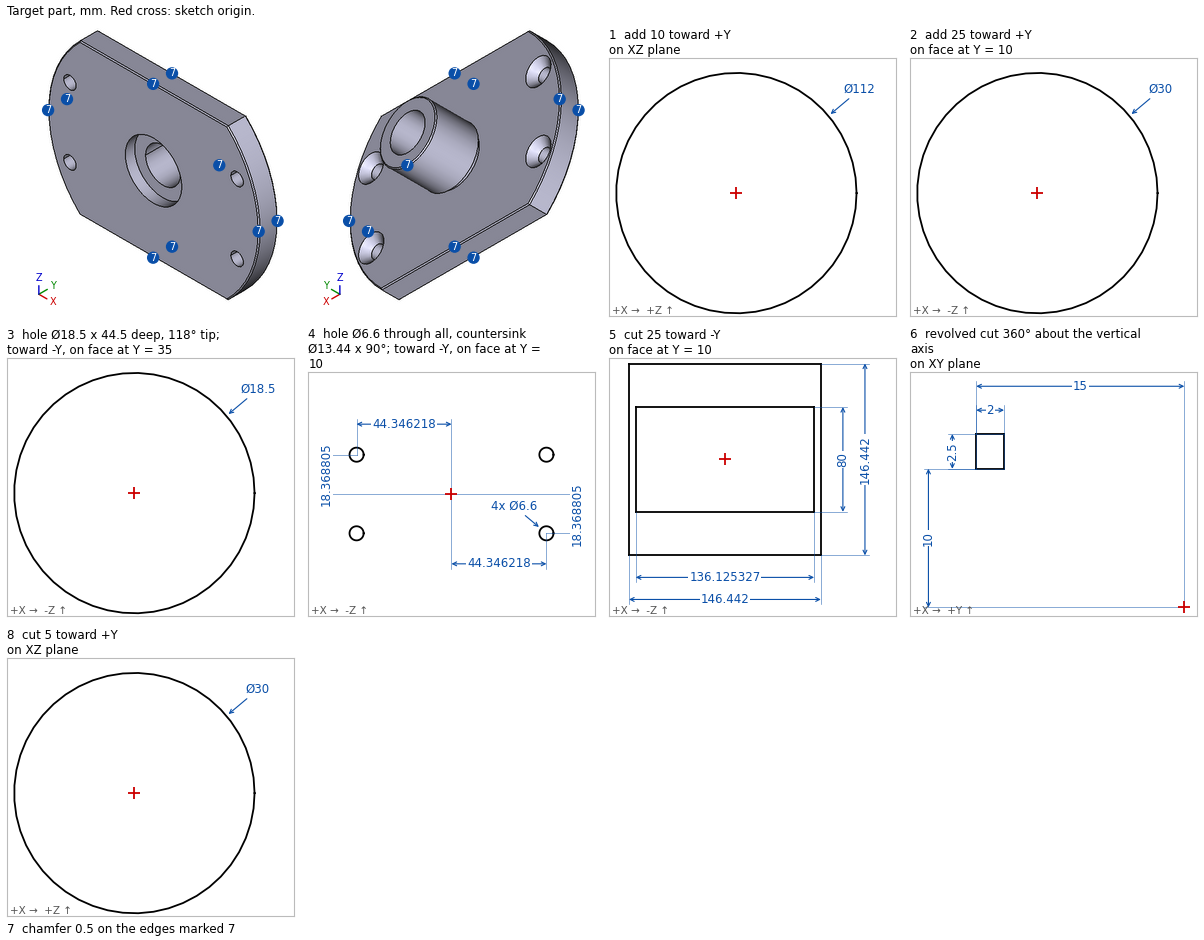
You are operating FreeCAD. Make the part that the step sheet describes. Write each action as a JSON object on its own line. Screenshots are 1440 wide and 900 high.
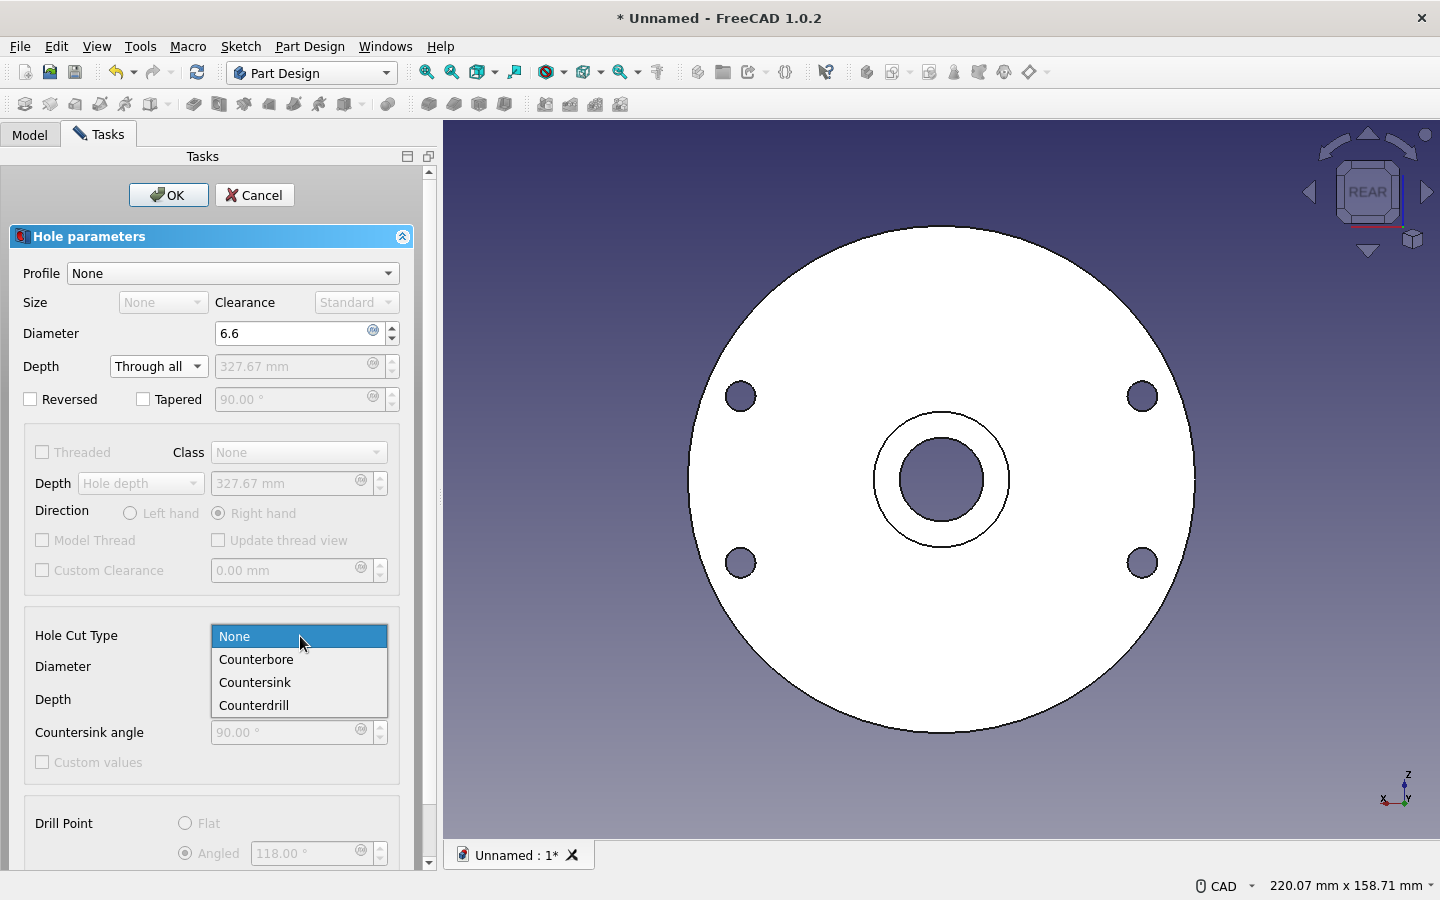
{"action": "left_click", "coordinate": [298, 682]}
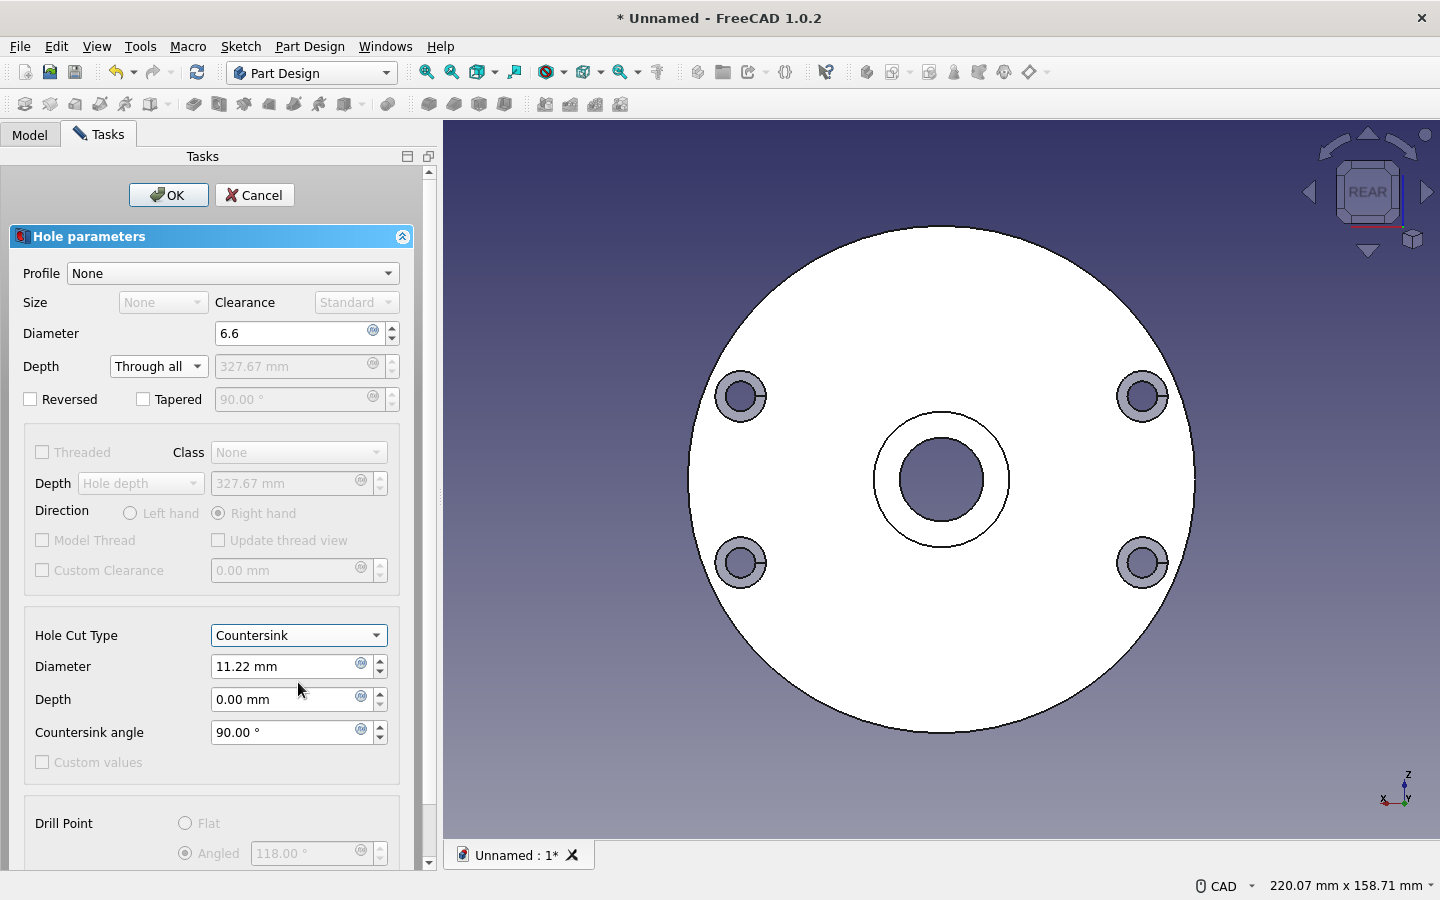
{"action": "triple_click", "coordinate": [292, 666]}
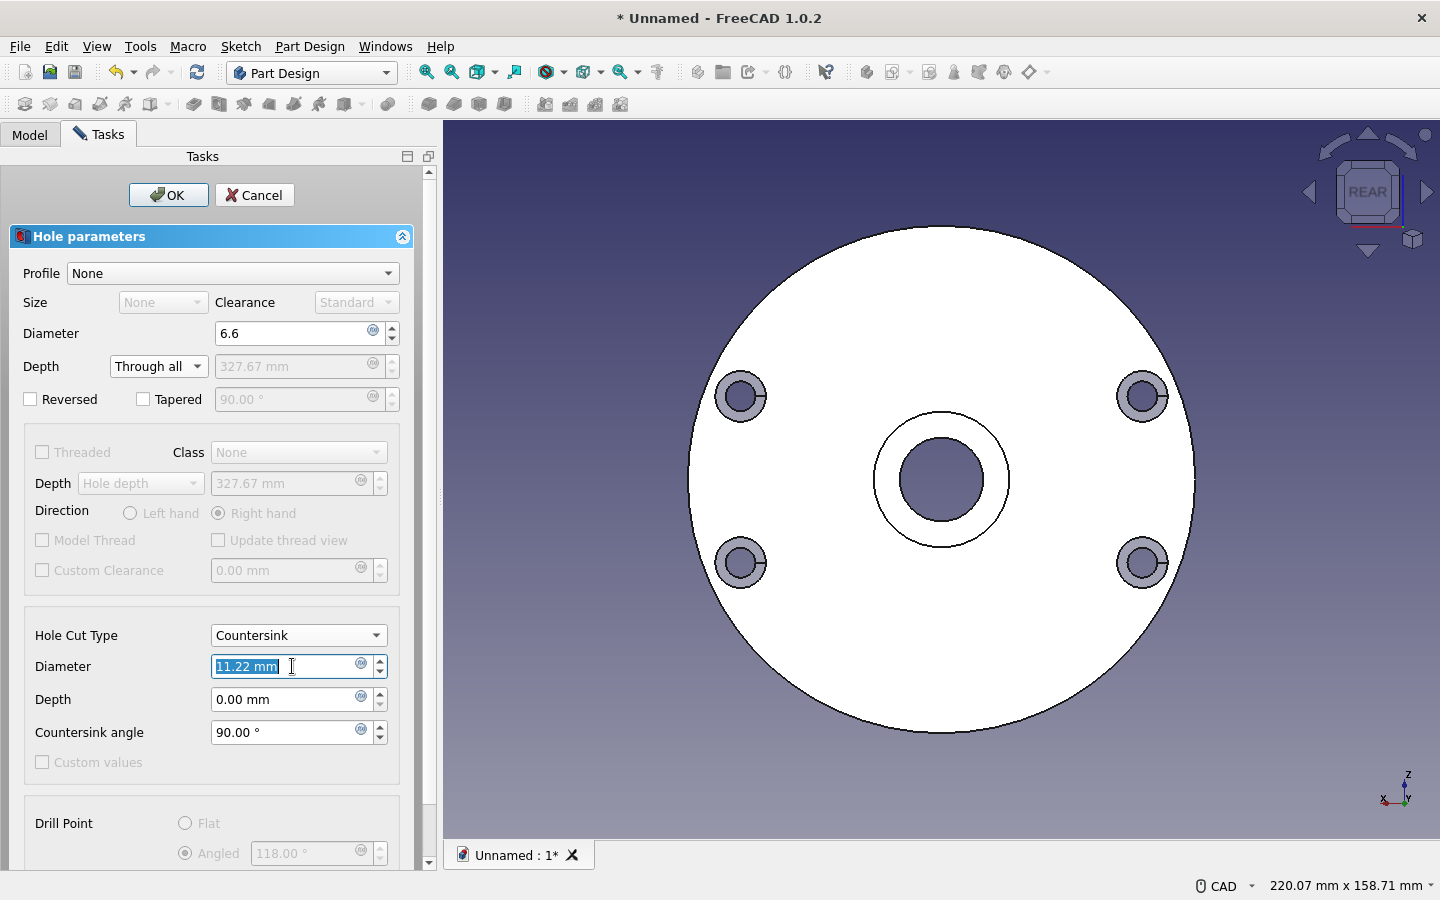
{"action": "type", "text": "13.44"}
{"action": "key", "text": "Tab"}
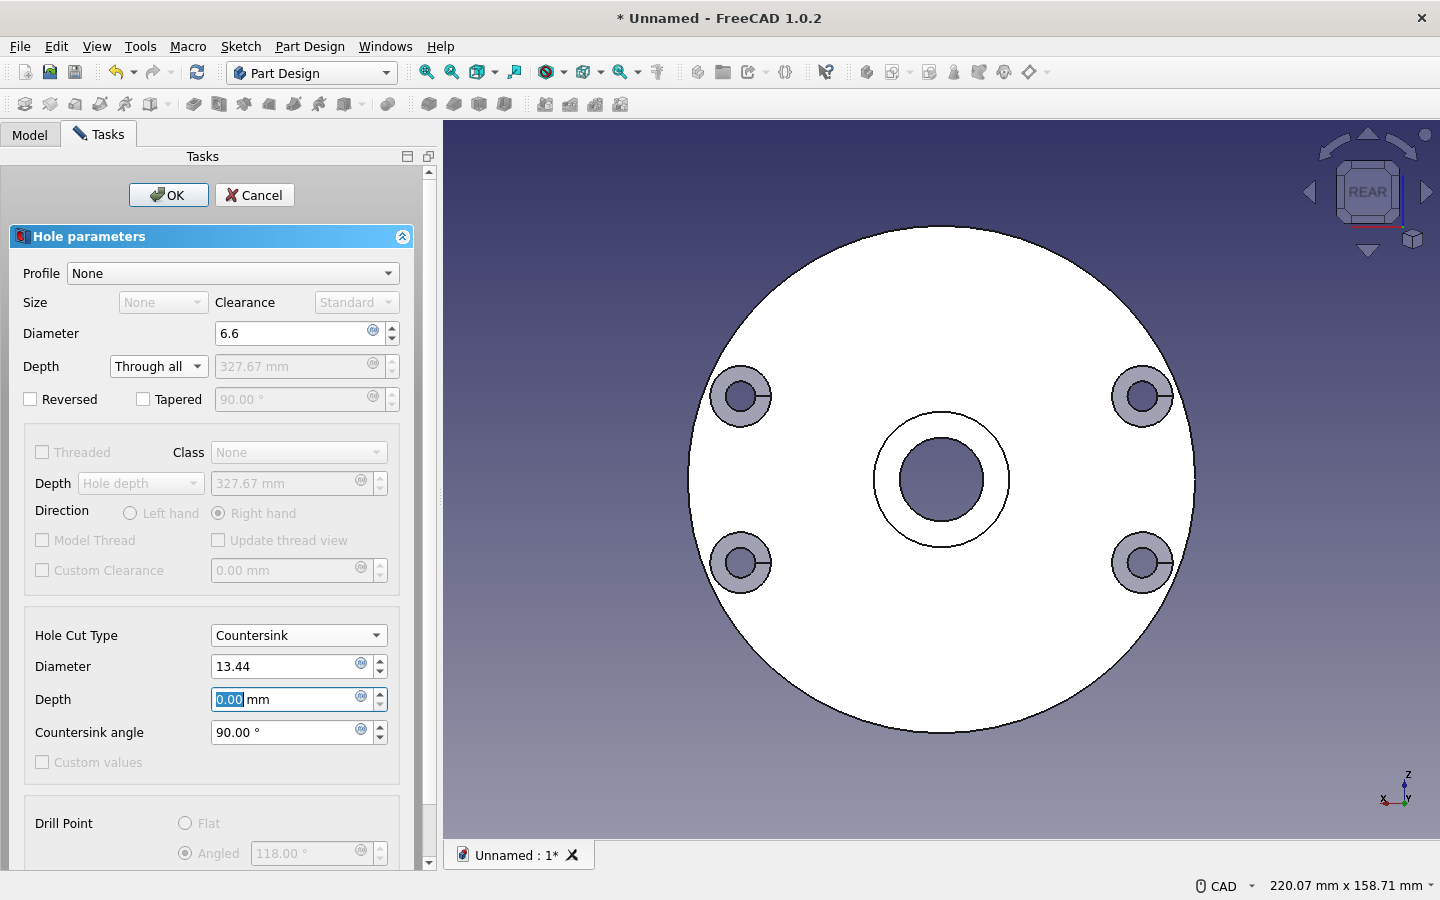
{"action": "left_click", "coordinate": [169, 195]}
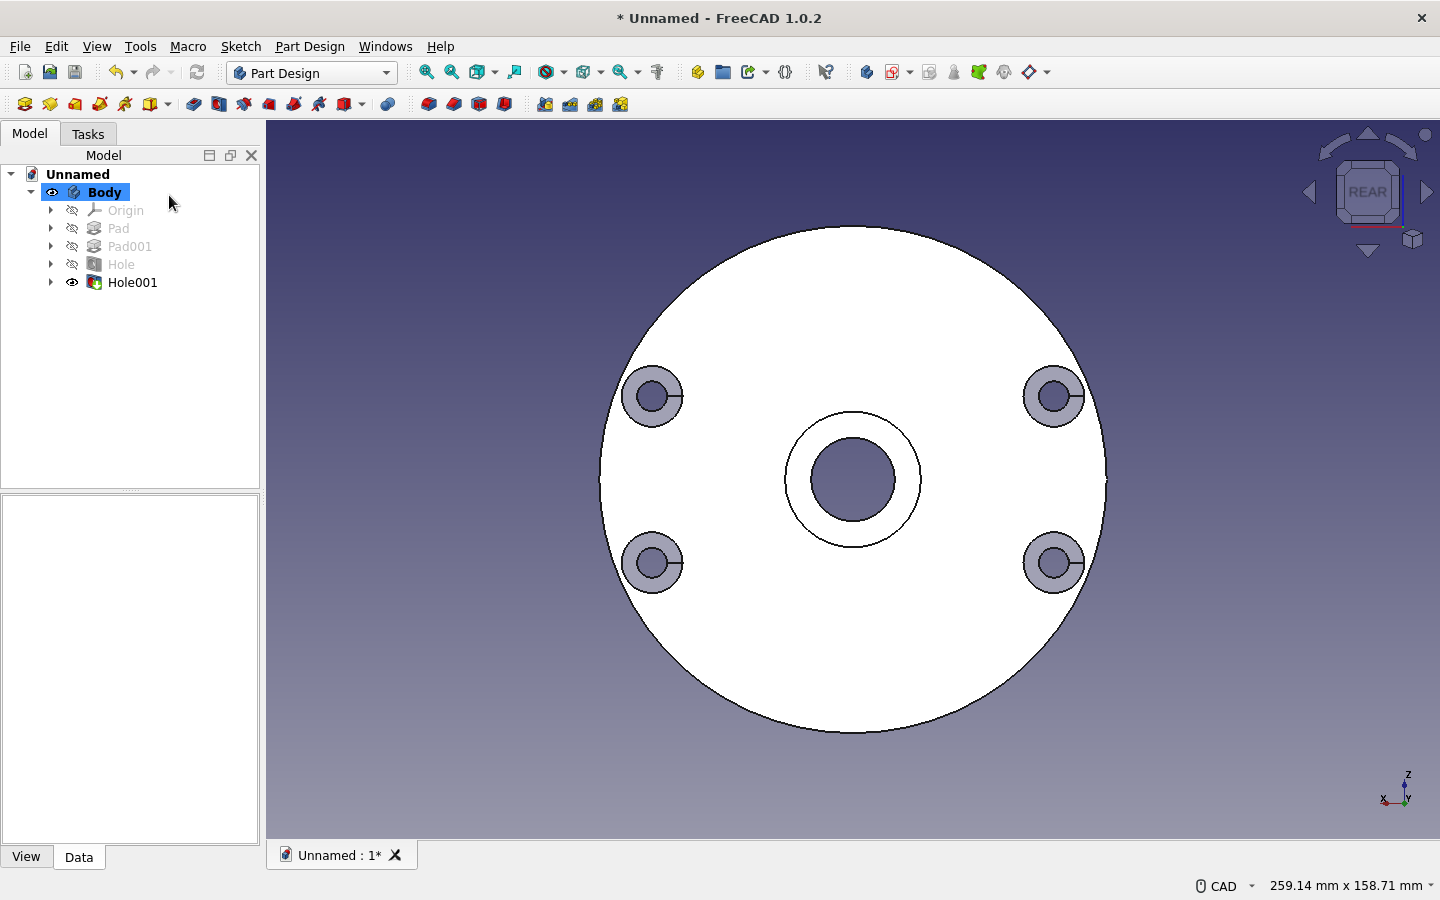
{"action": "left_click", "coordinate": [781, 334]}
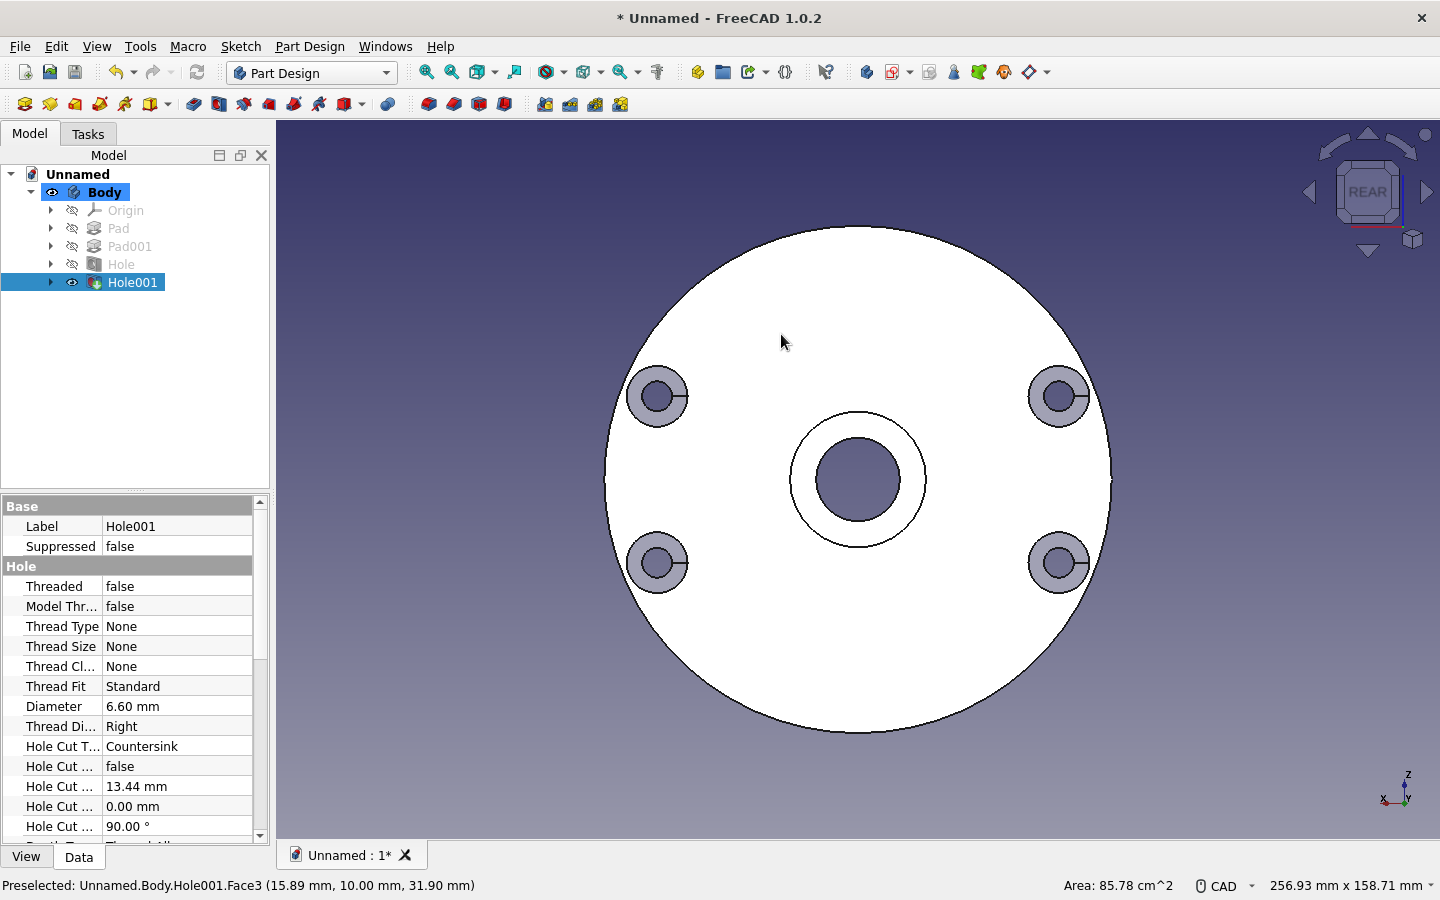
{"action": "left_click", "coordinate": [892, 72]}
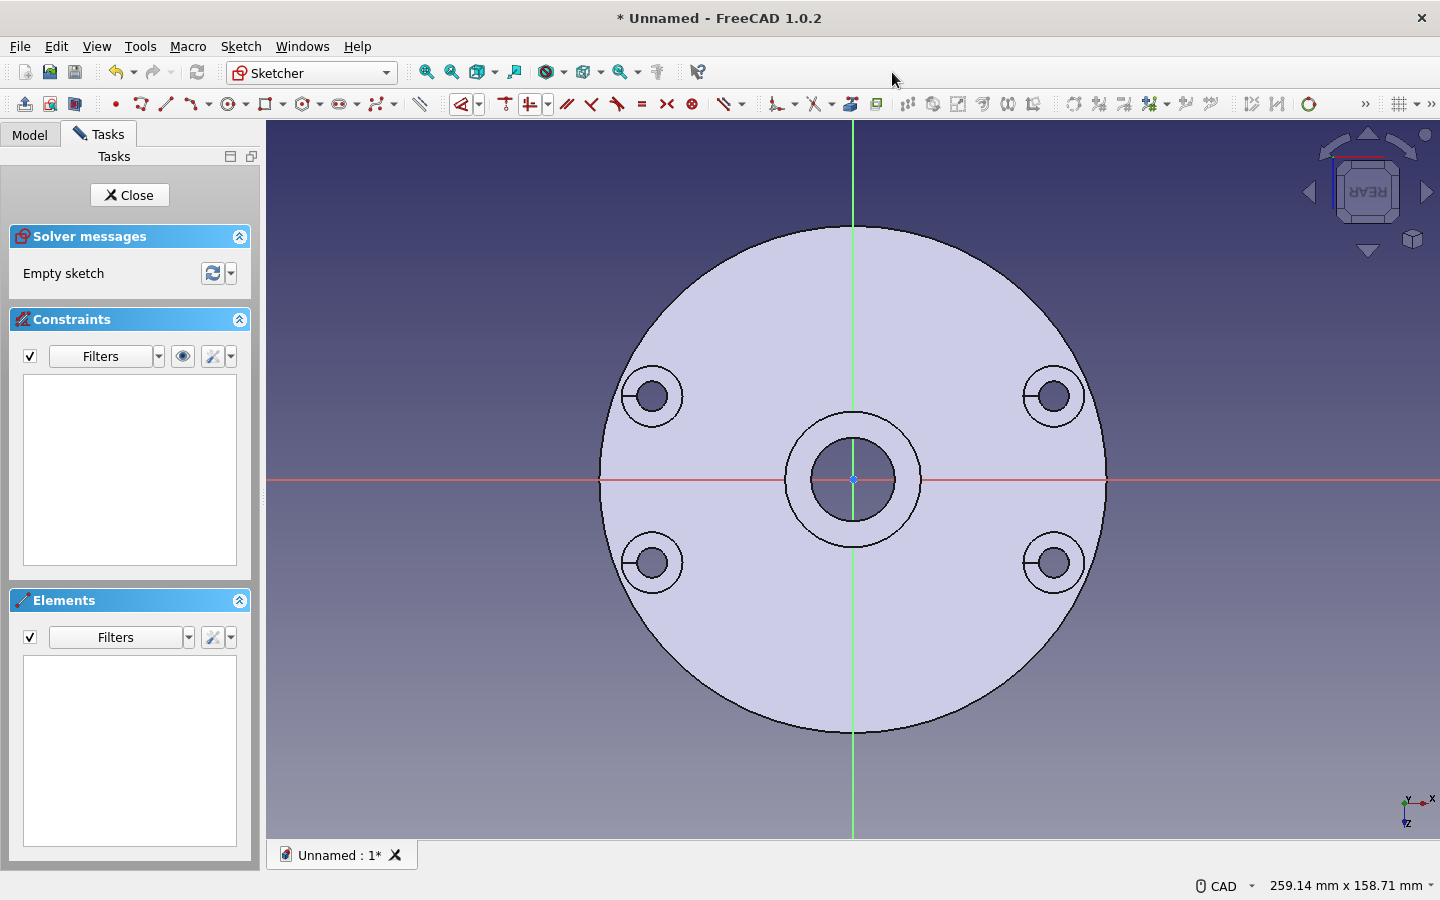
{"action": "key", "text": "q s"}